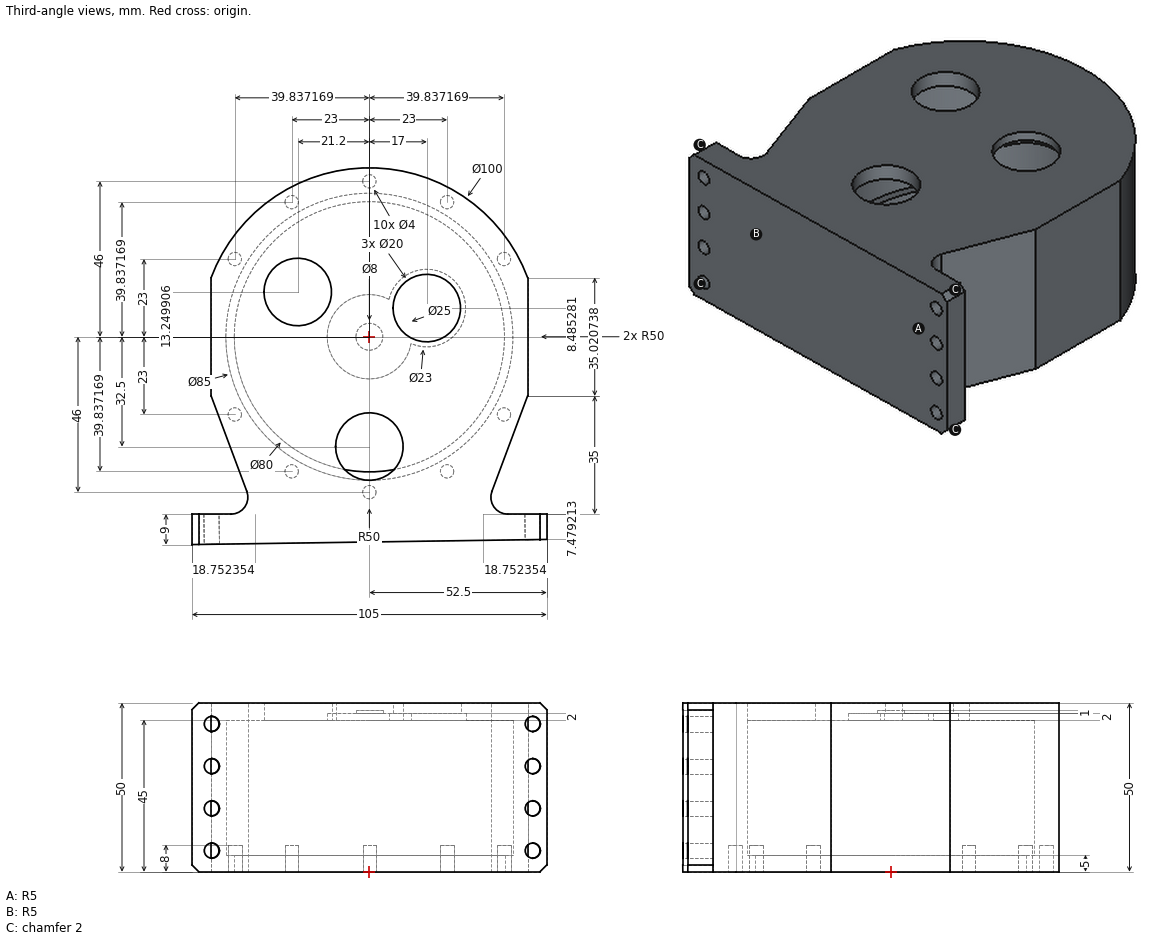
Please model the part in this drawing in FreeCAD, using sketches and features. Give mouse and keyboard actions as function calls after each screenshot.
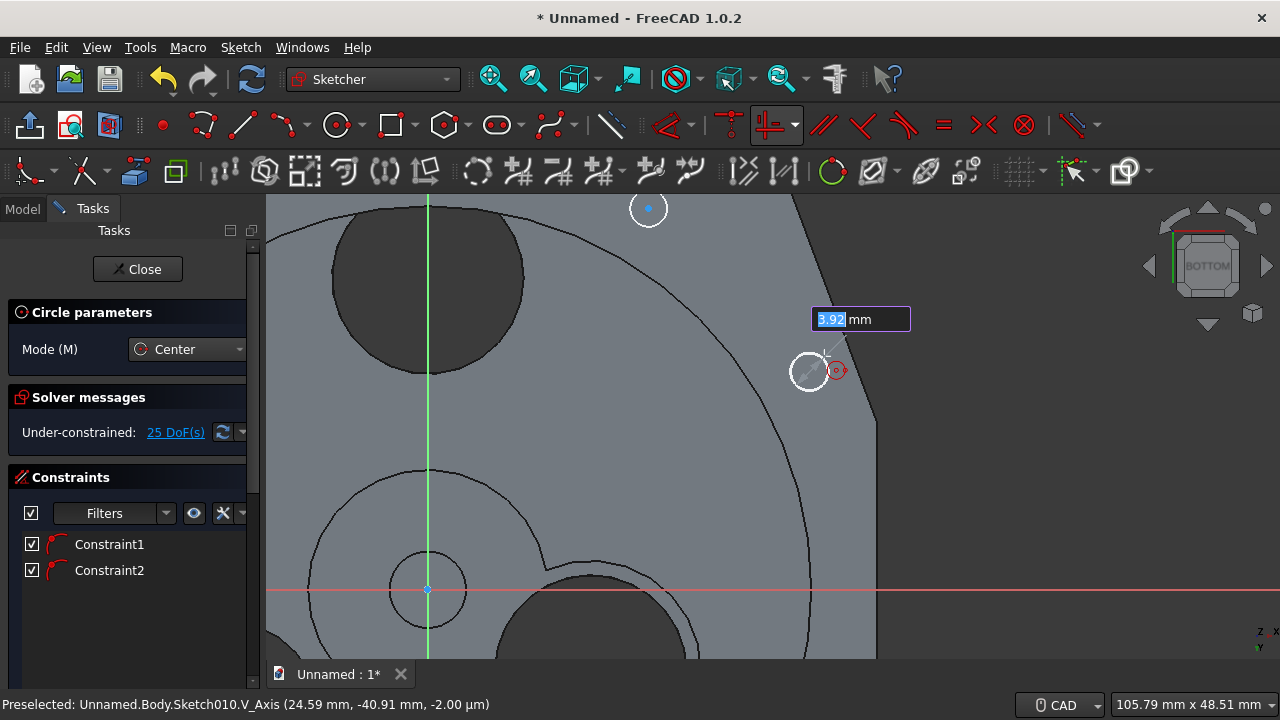
click(823, 356)
key(Escape)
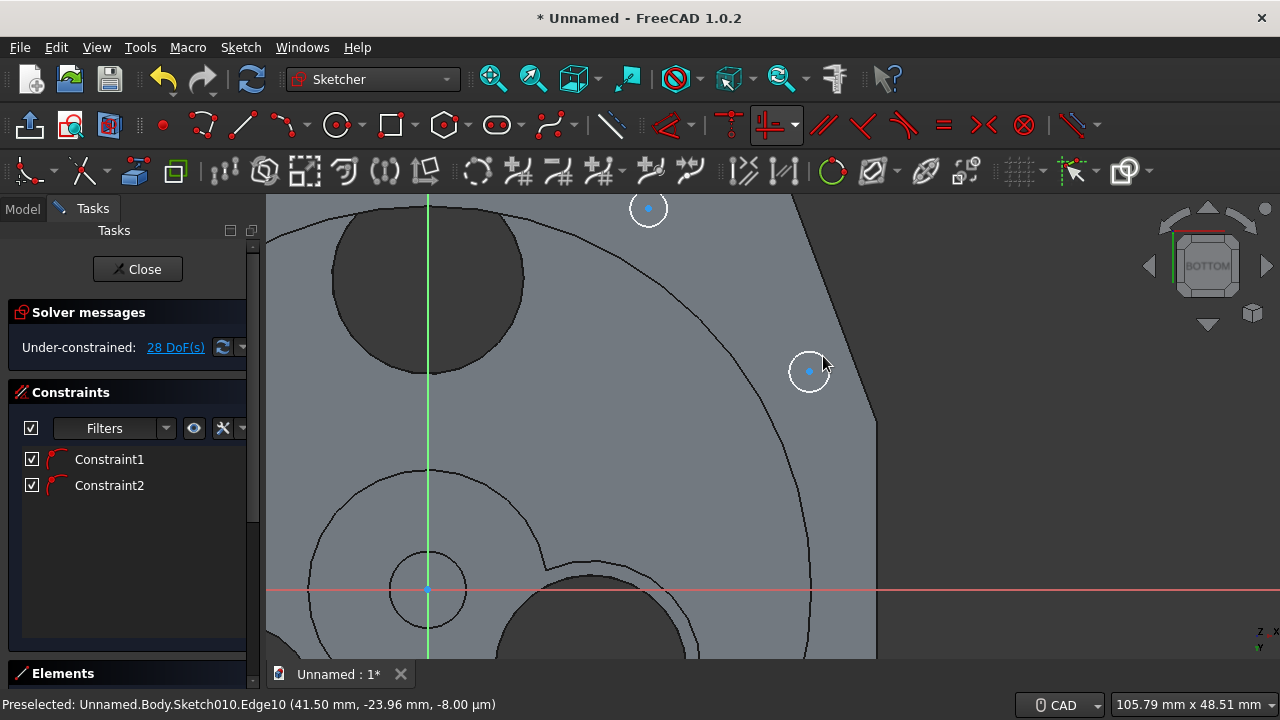
scroll(824, 356, down, 6)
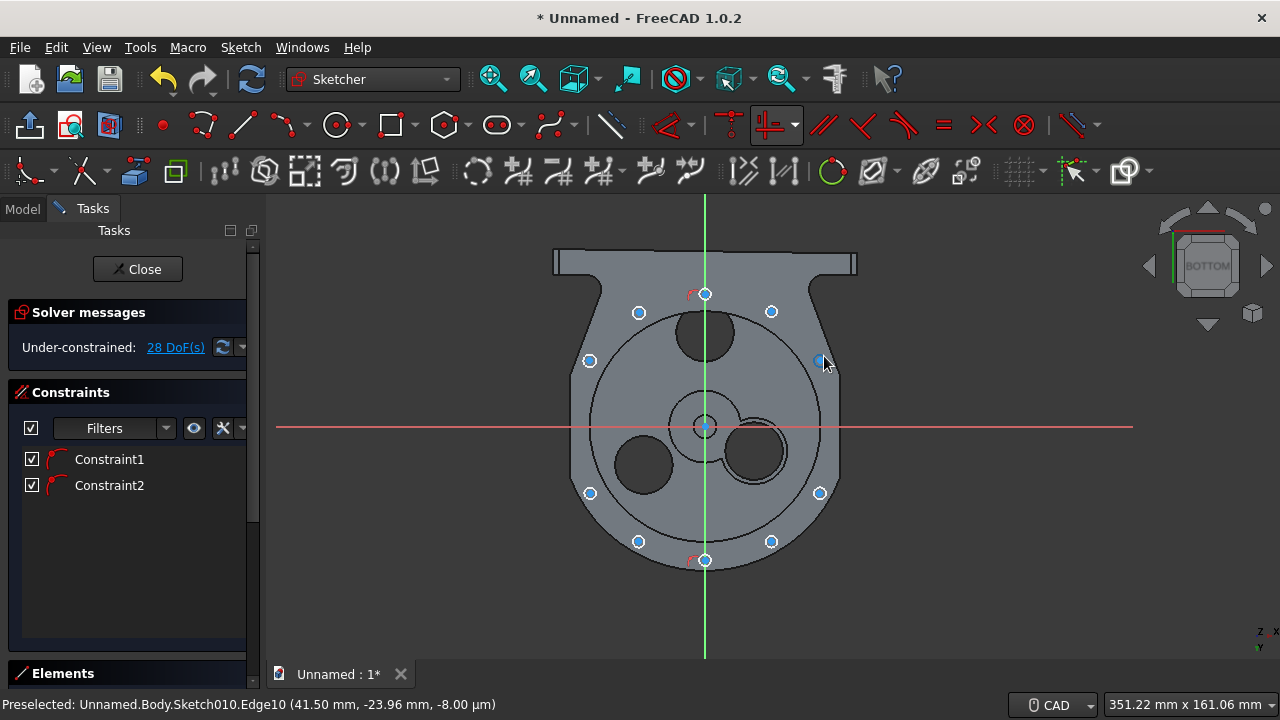
scroll(709, 556, up, 7)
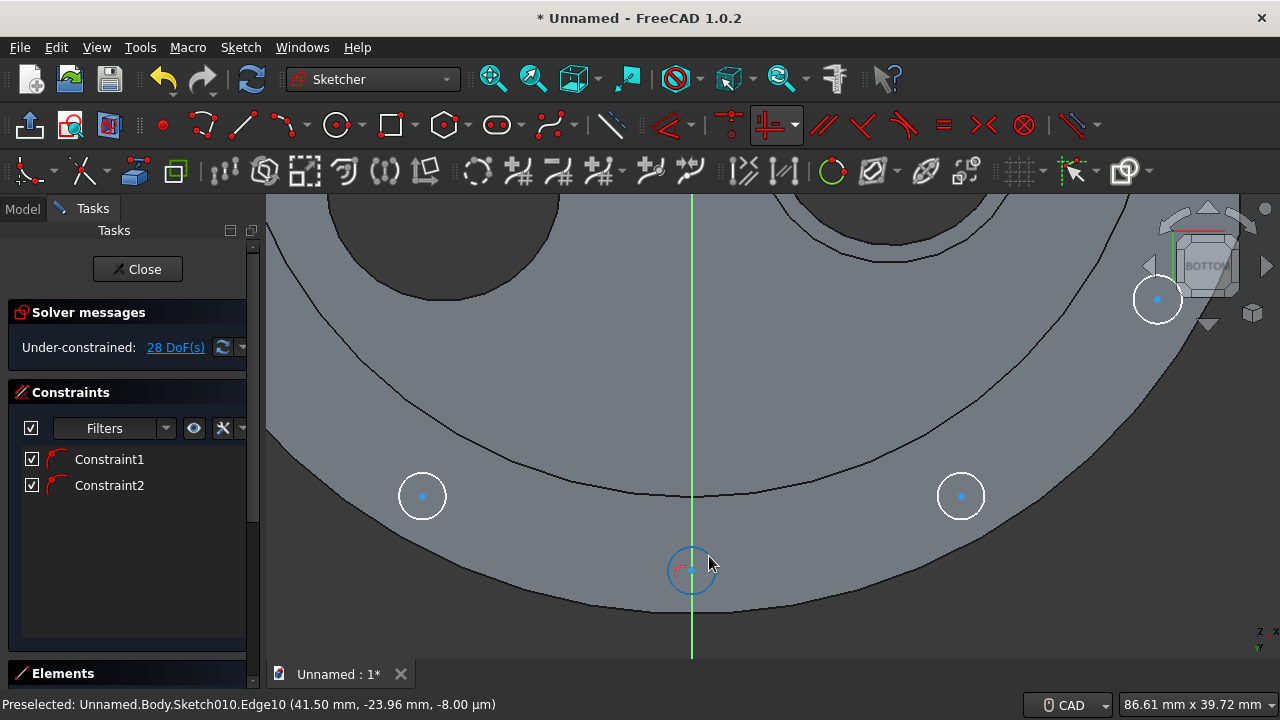
click(708, 554)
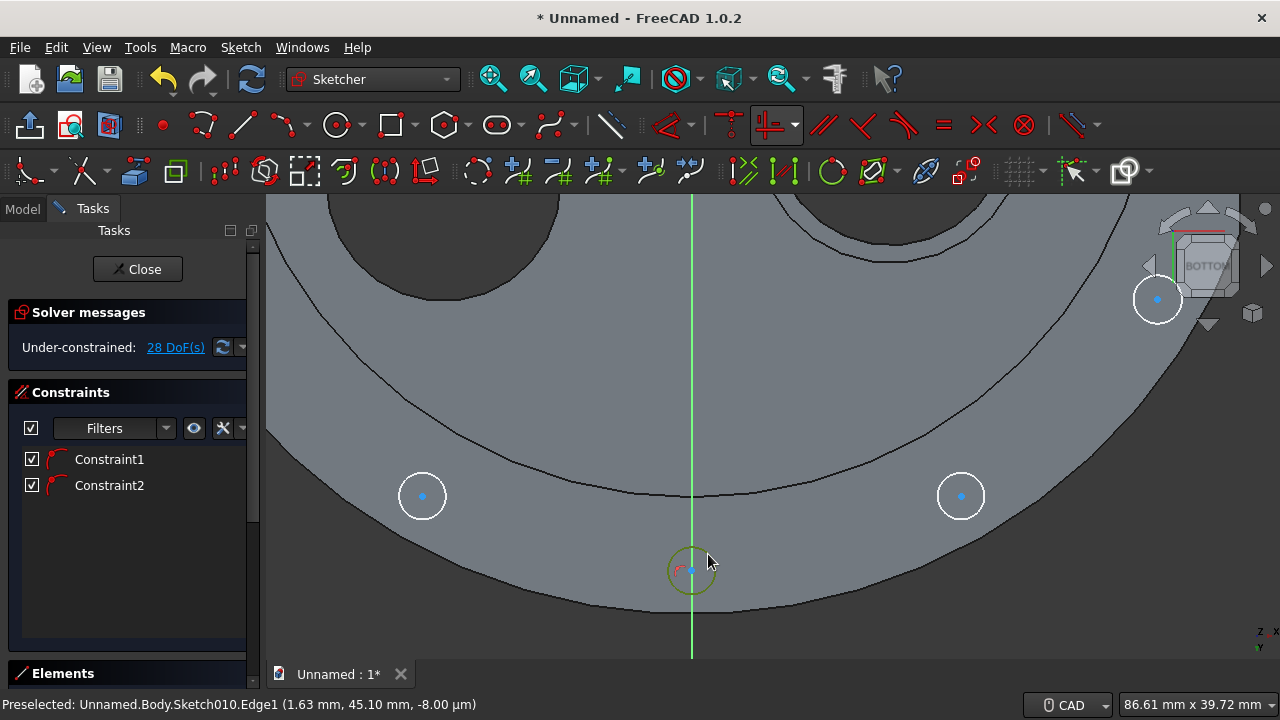
click(439, 480)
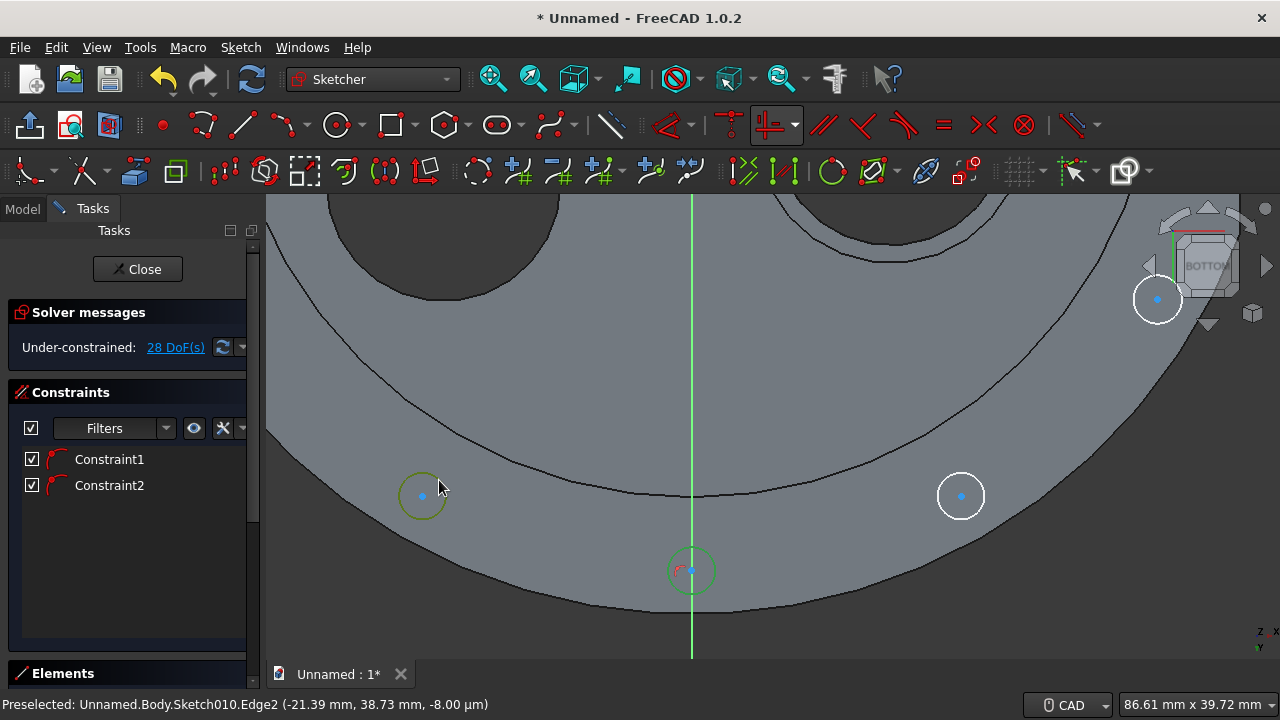
scroll(709, 557, down, 7)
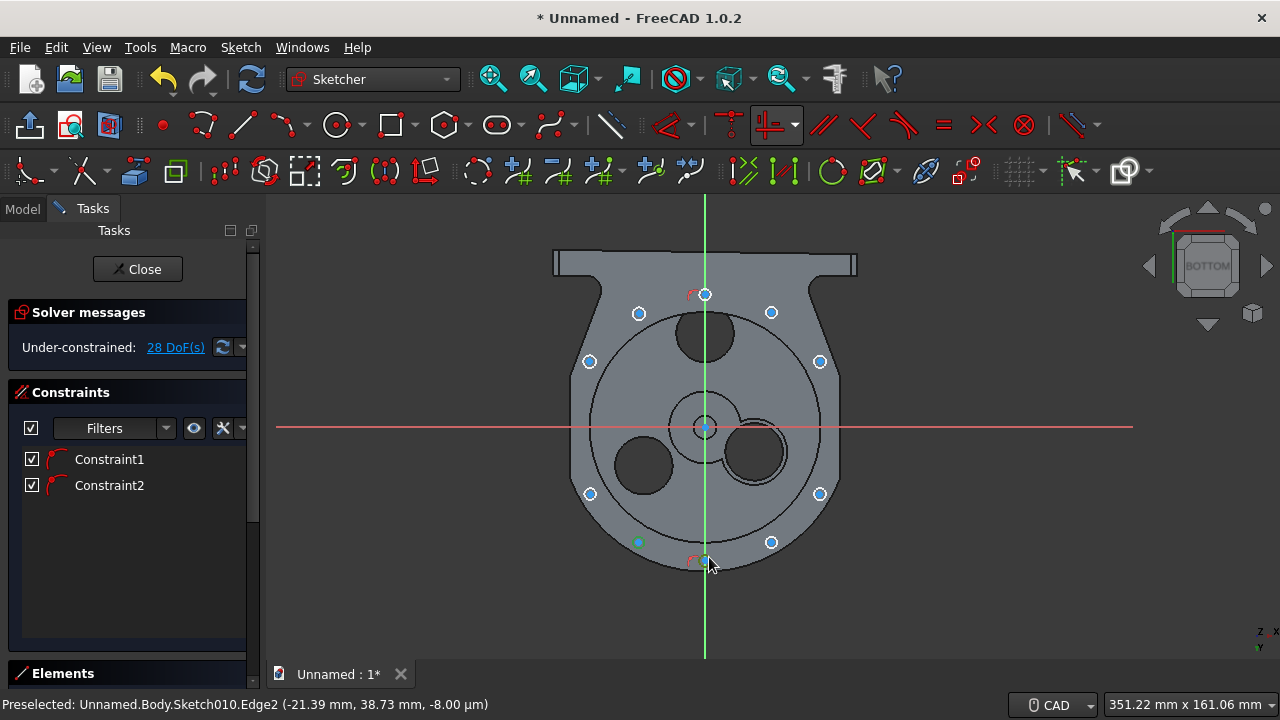
scroll(594, 490, up, 5)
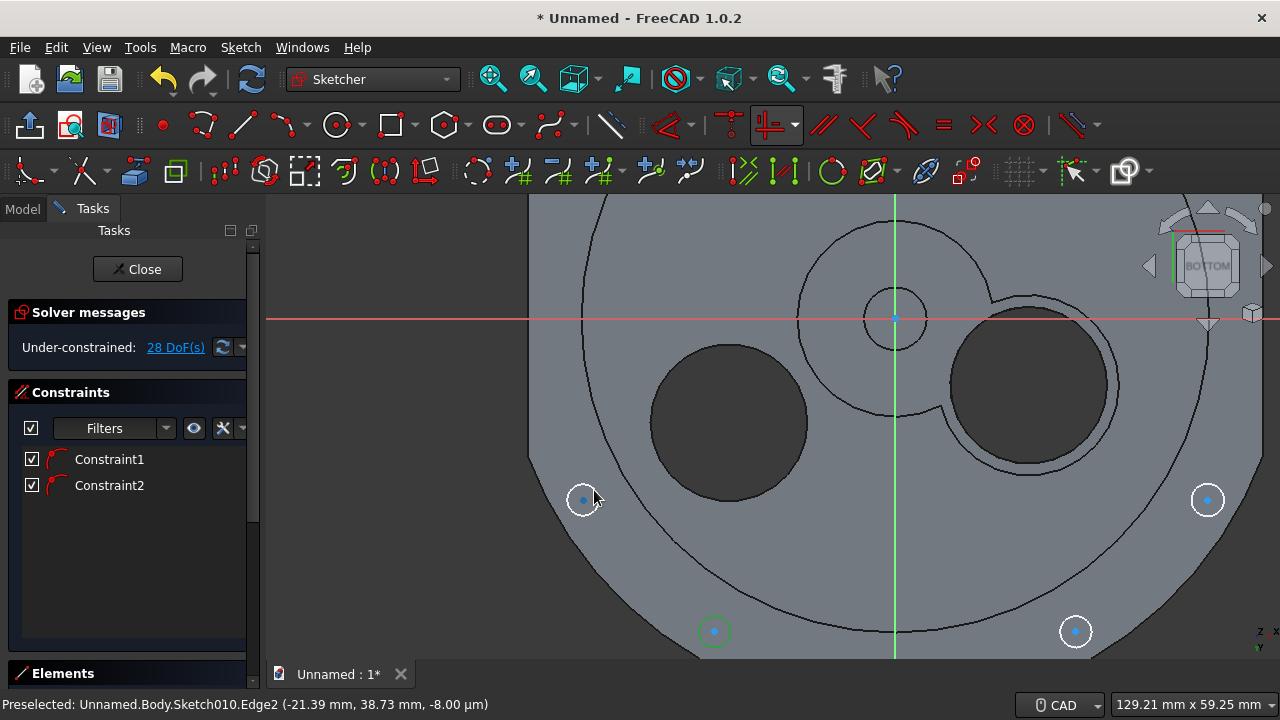
click(594, 489)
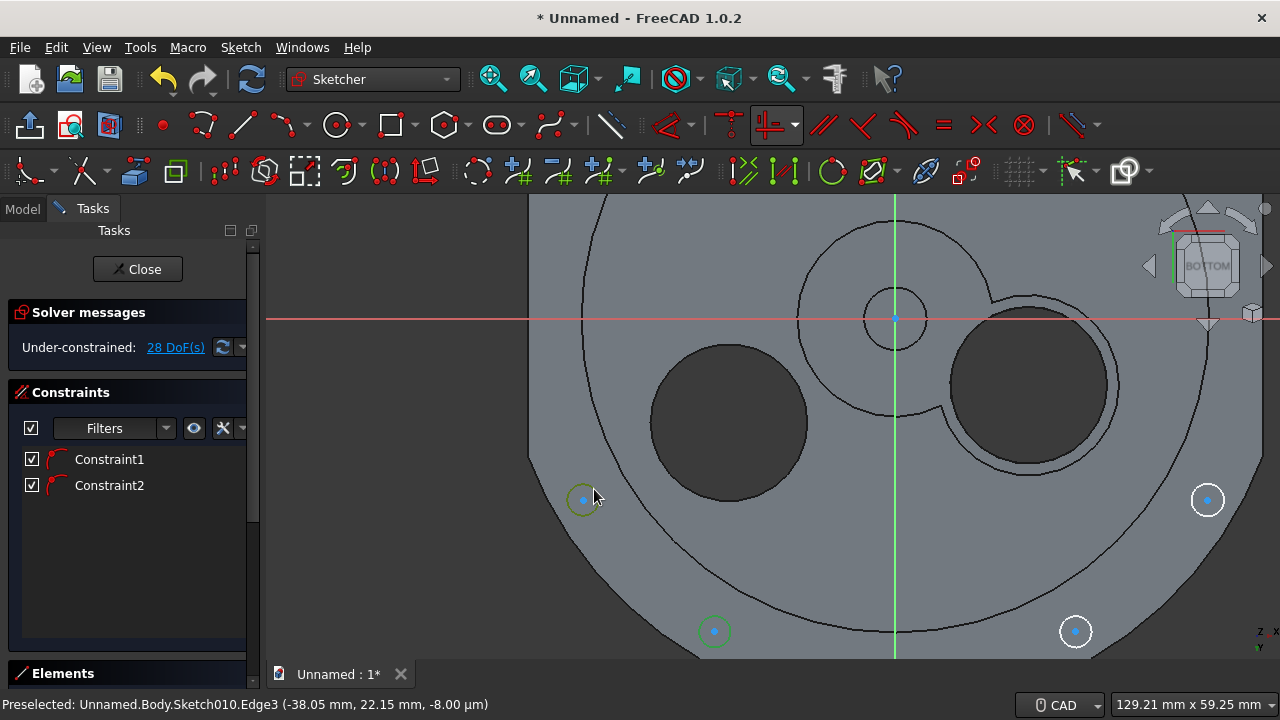
click(1087, 621)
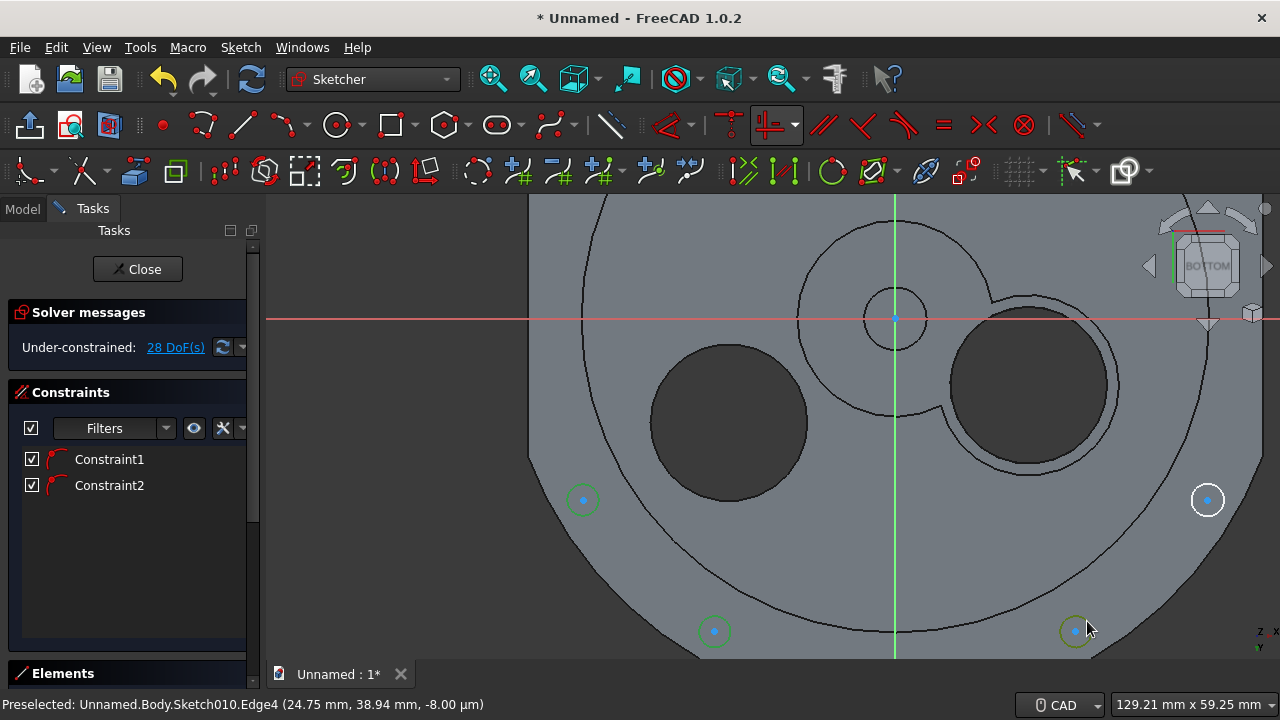
scroll(593, 489, down, 5)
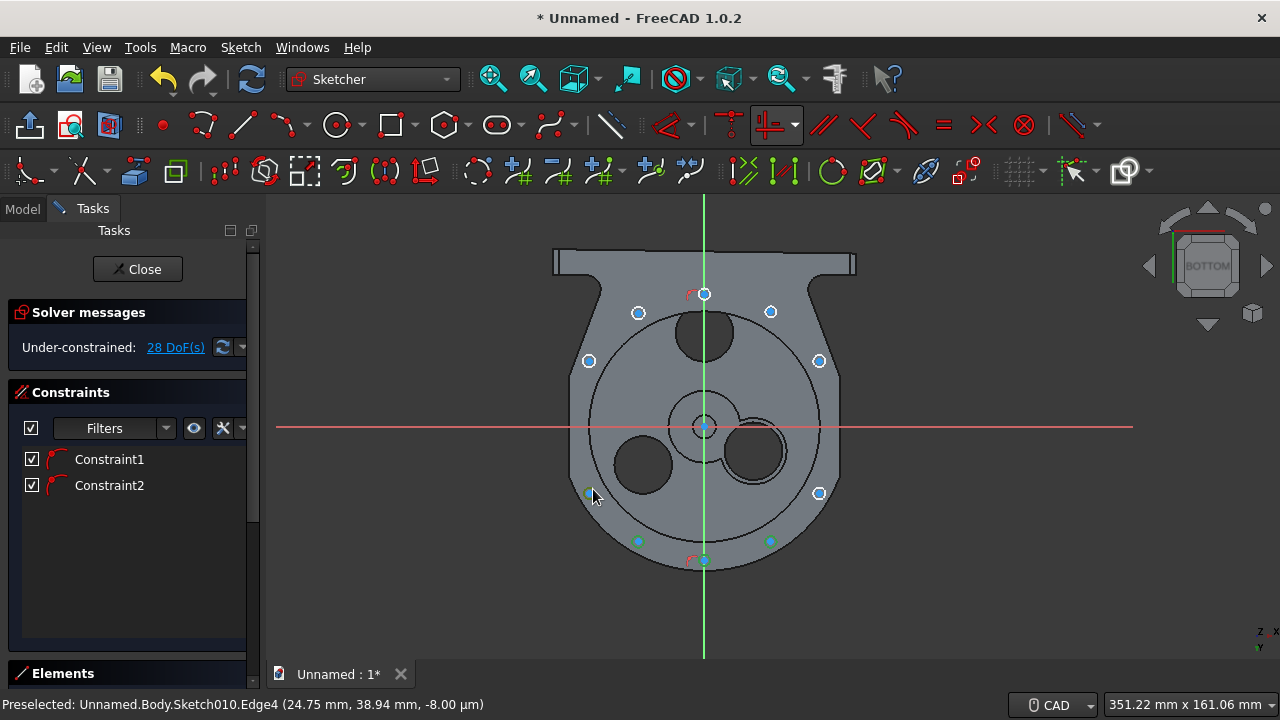
scroll(824, 489, up, 5)